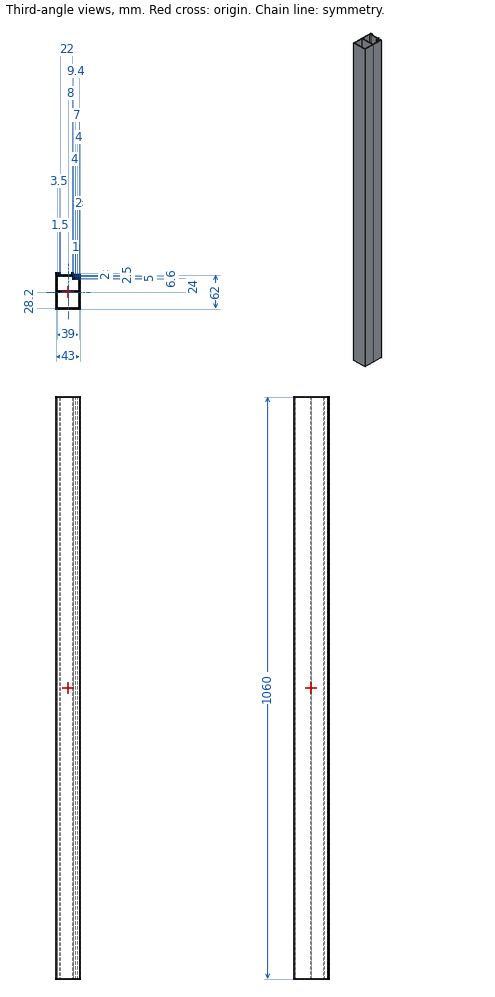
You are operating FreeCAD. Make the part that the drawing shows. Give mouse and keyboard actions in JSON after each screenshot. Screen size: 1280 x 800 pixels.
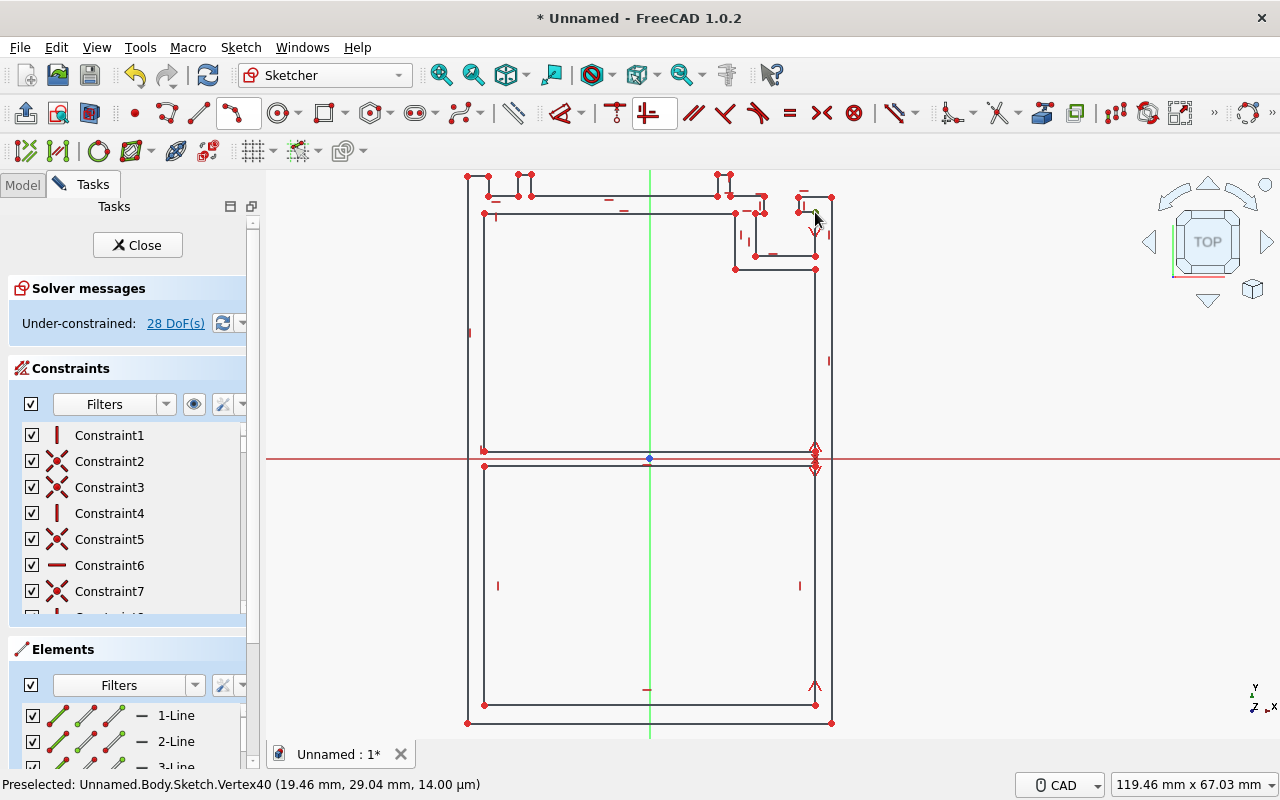
{"action": "left_click", "coordinate": [484, 214]}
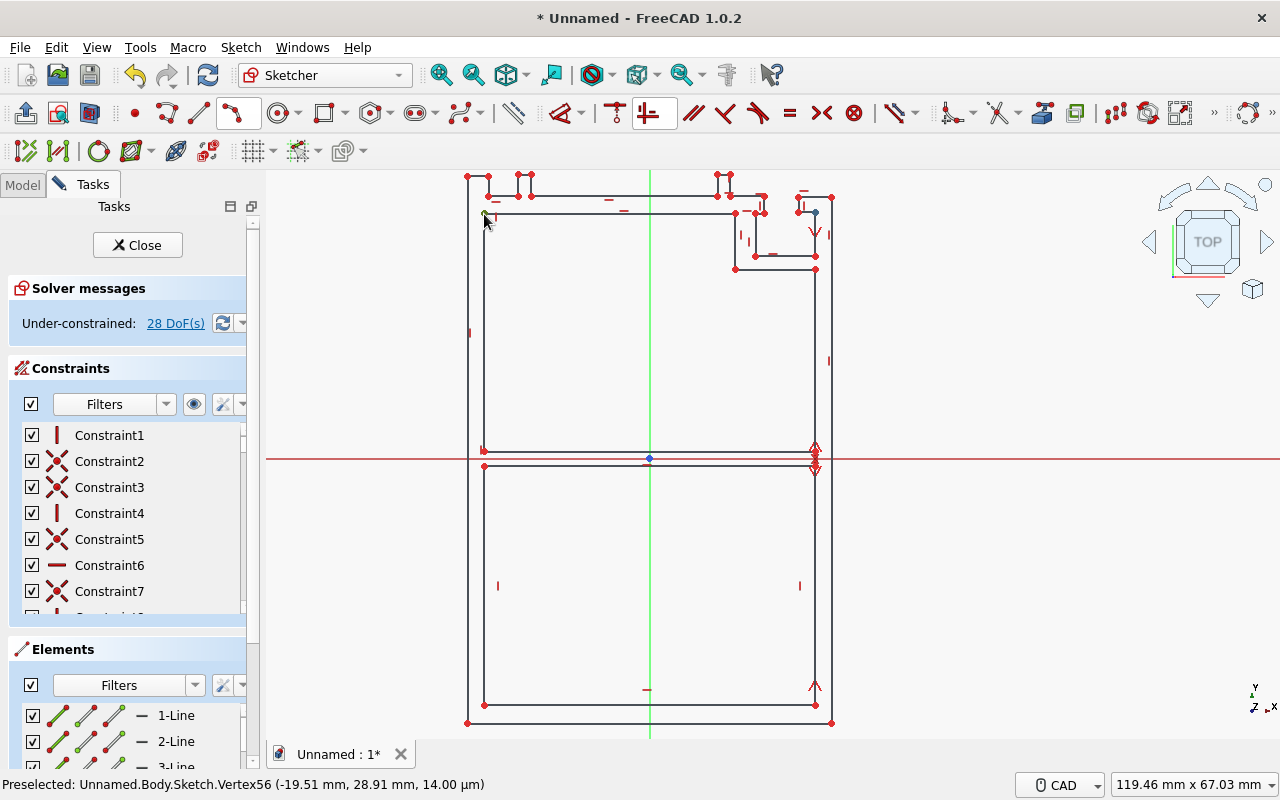
{"action": "left_click", "coordinate": [650, 674]}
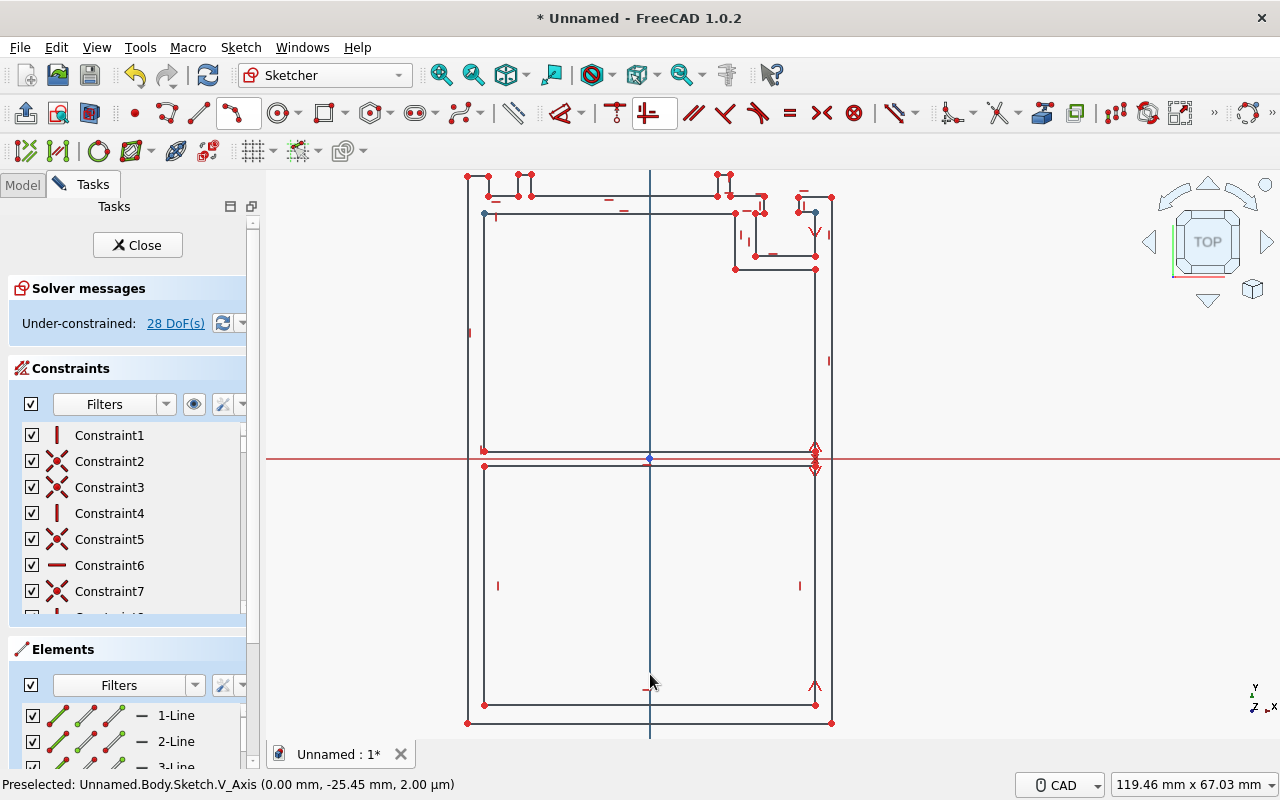
{"action": "left_click", "coordinate": [822, 114]}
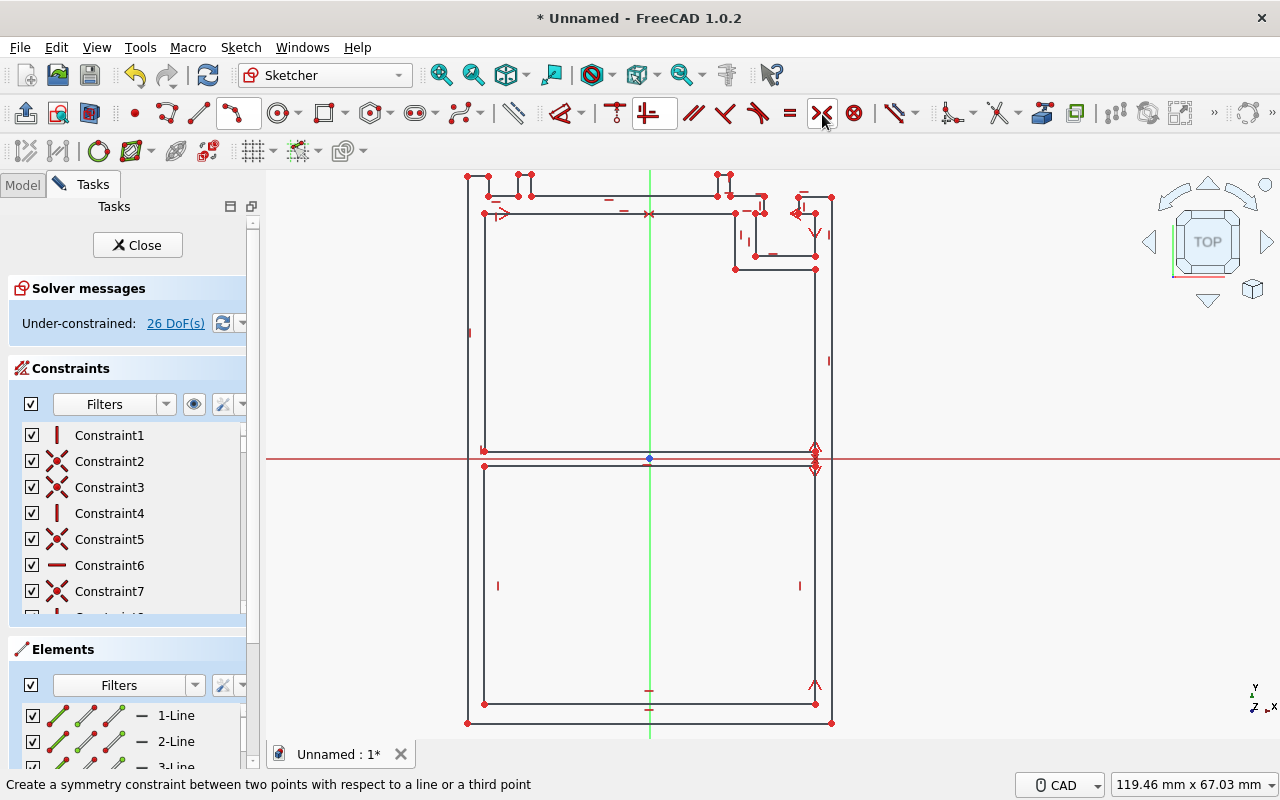
{"action": "left_click", "coordinate": [756, 243]}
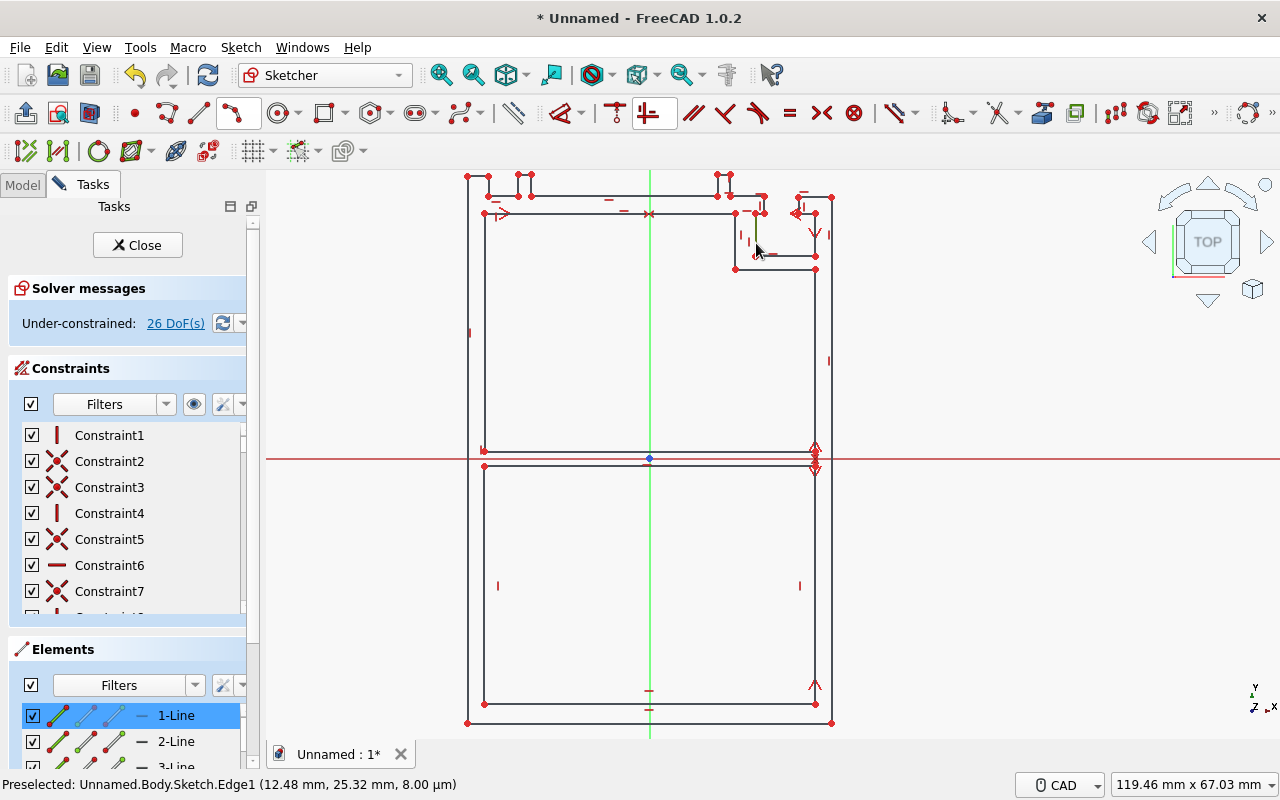
{"action": "left_click", "coordinate": [584, 114]}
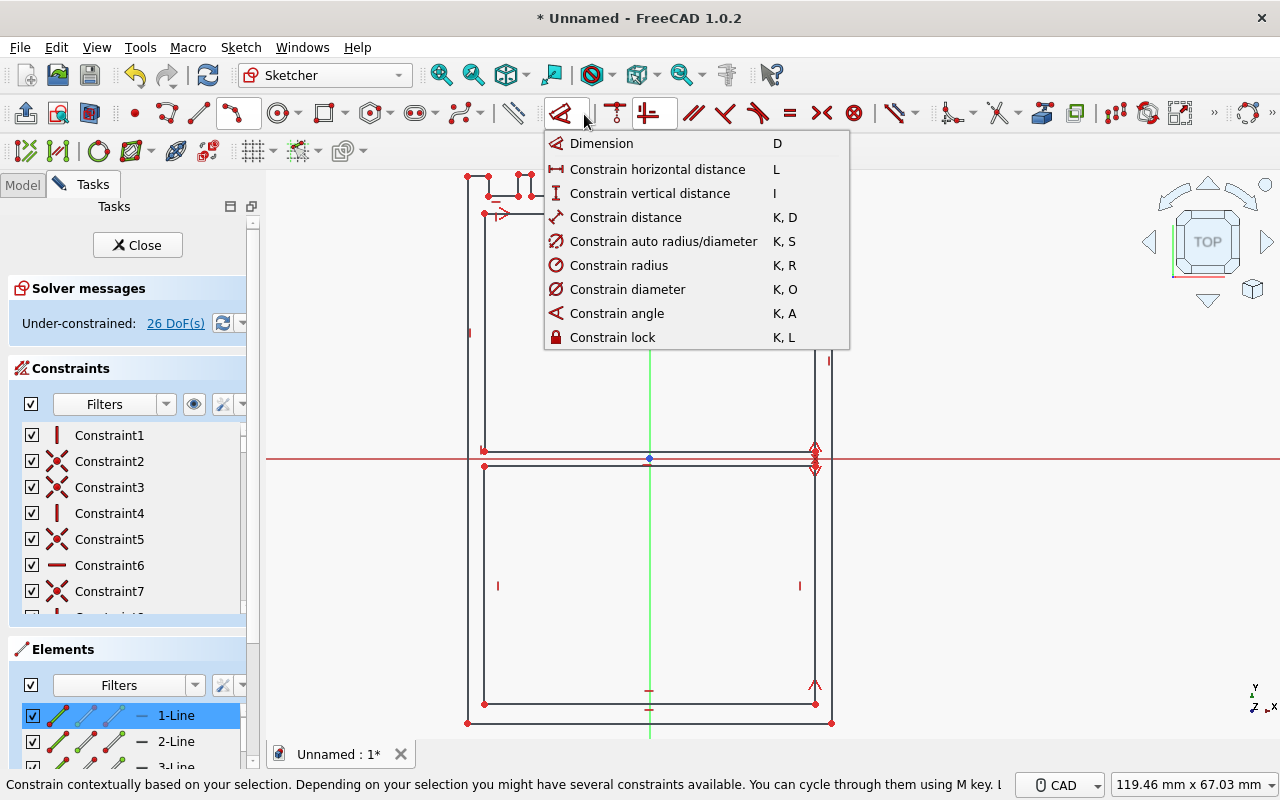
{"action": "left_click", "coordinate": [697, 193]}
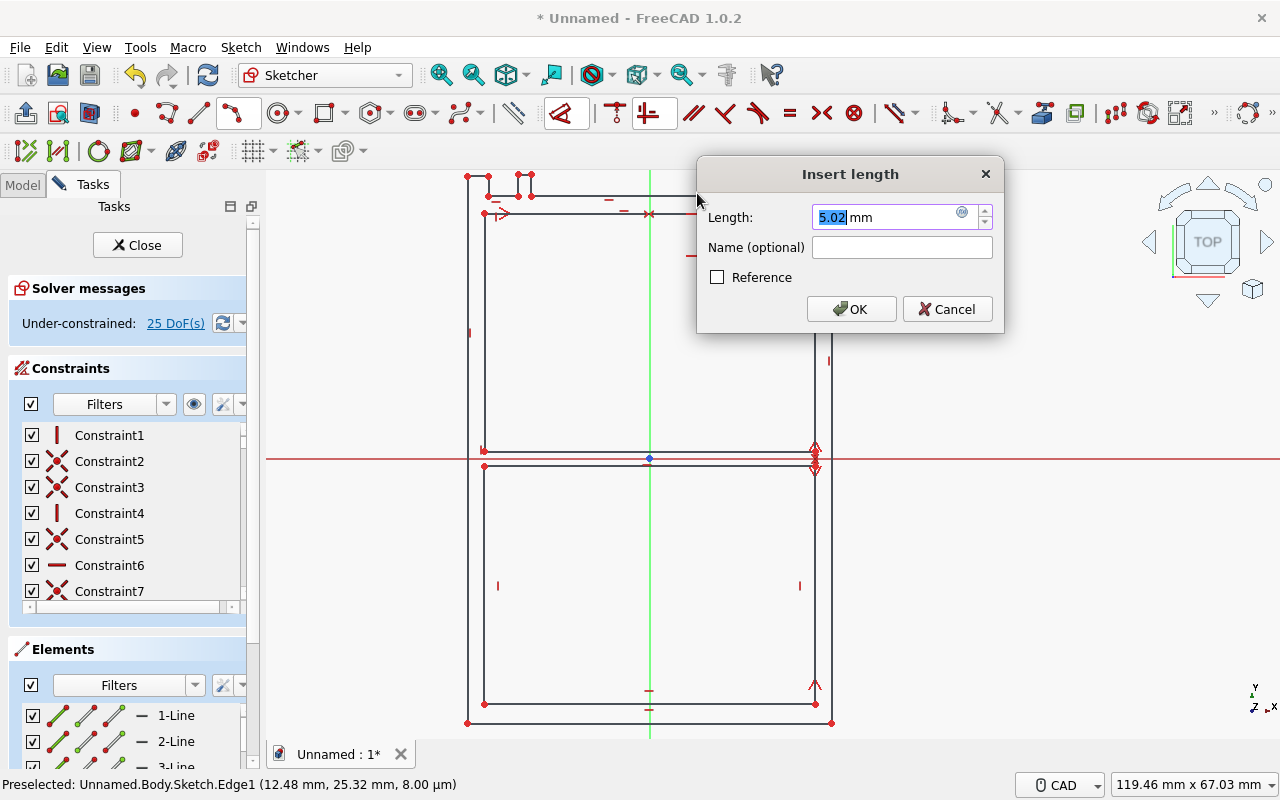
{"action": "type", "text": "5"}
{"action": "key", "text": "Return"}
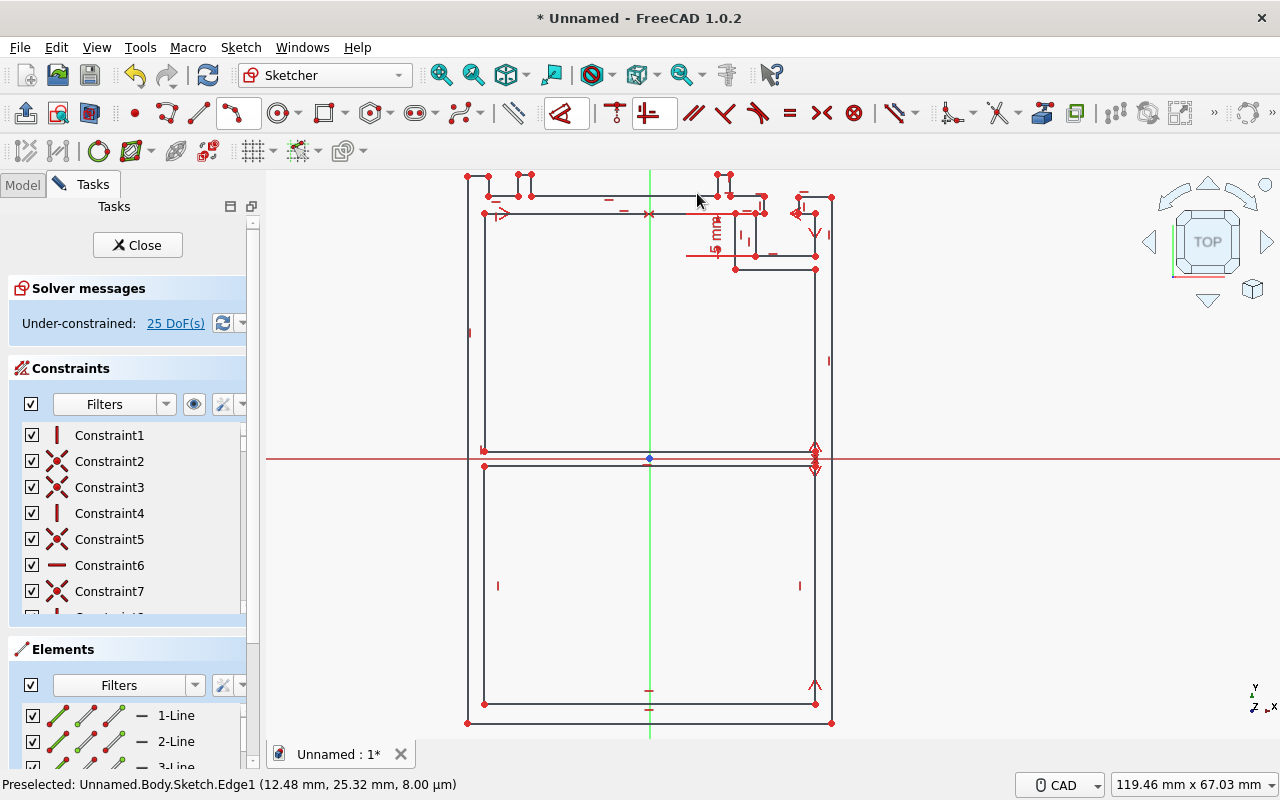
{"action": "scroll", "coordinate": [760, 214], "scroll_direction": "up", "scroll_amount": 8}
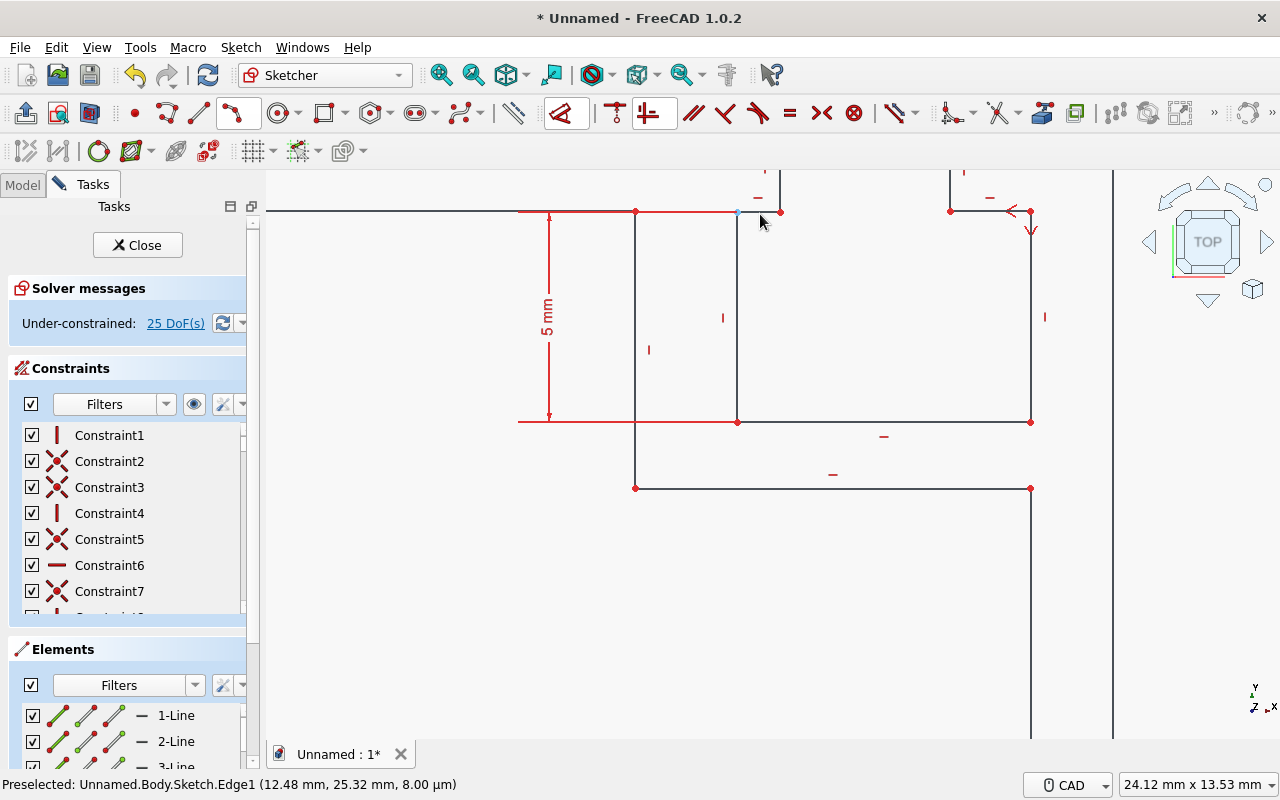
{"action": "left_click", "coordinate": [759, 212]}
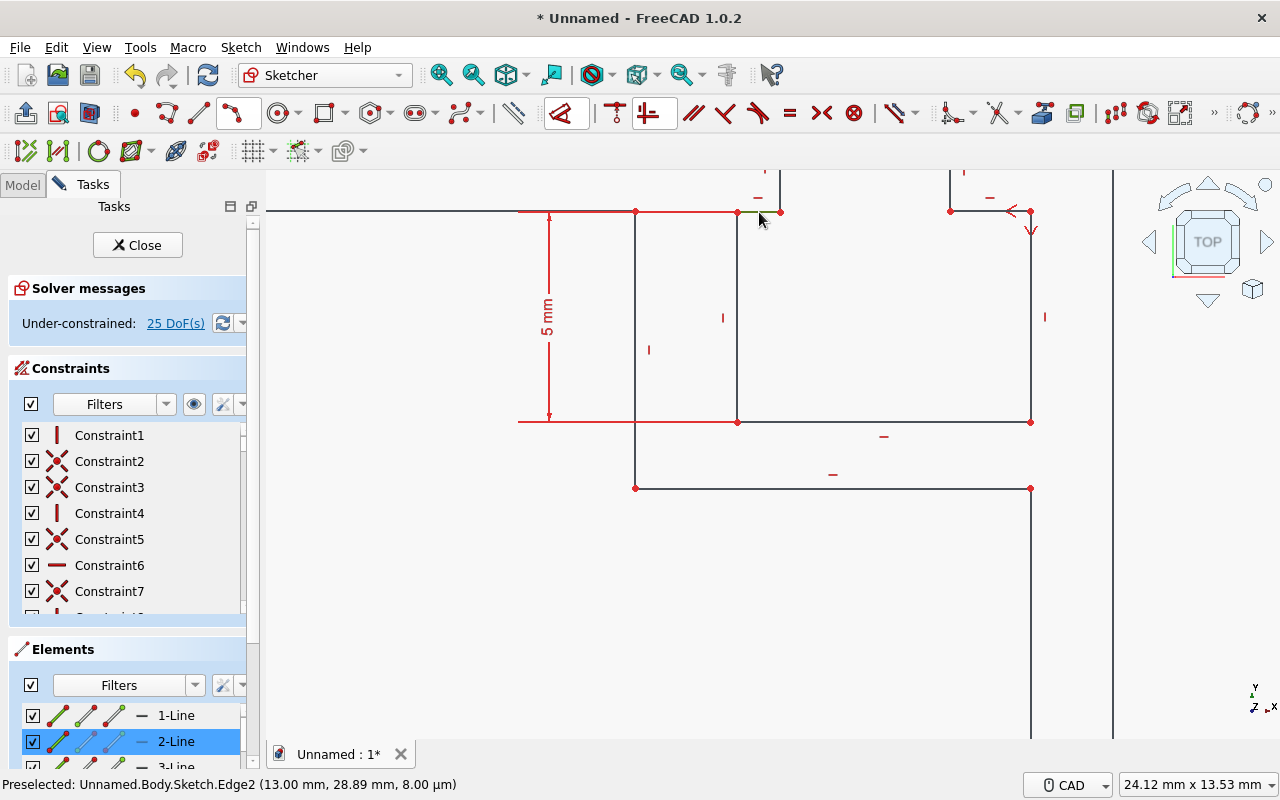
{"action": "left_click", "coordinate": [584, 114]}